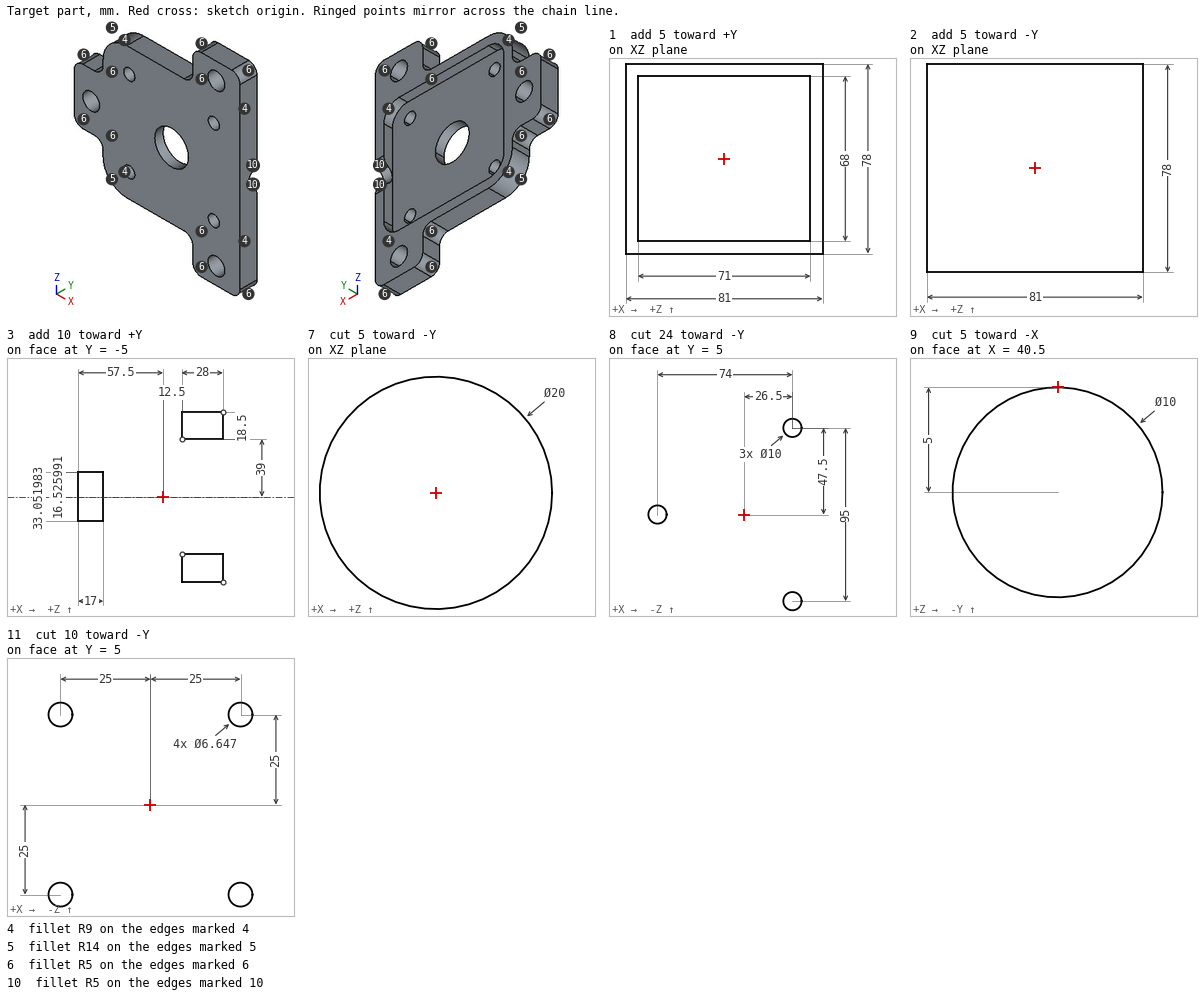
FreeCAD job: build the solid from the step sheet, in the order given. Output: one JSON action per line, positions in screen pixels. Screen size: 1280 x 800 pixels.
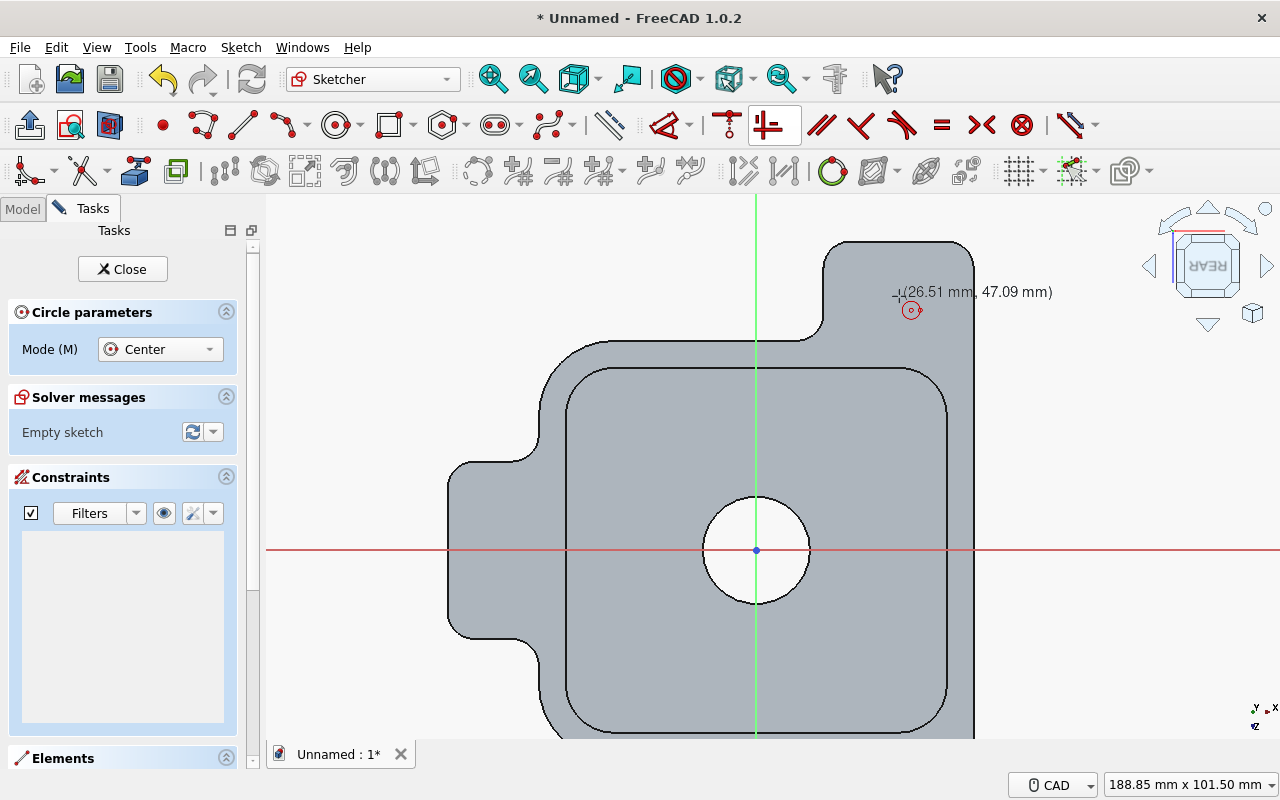
{"action": "left_click", "coordinate": [899, 295]}
{"action": "left_click", "coordinate": [918, 276]}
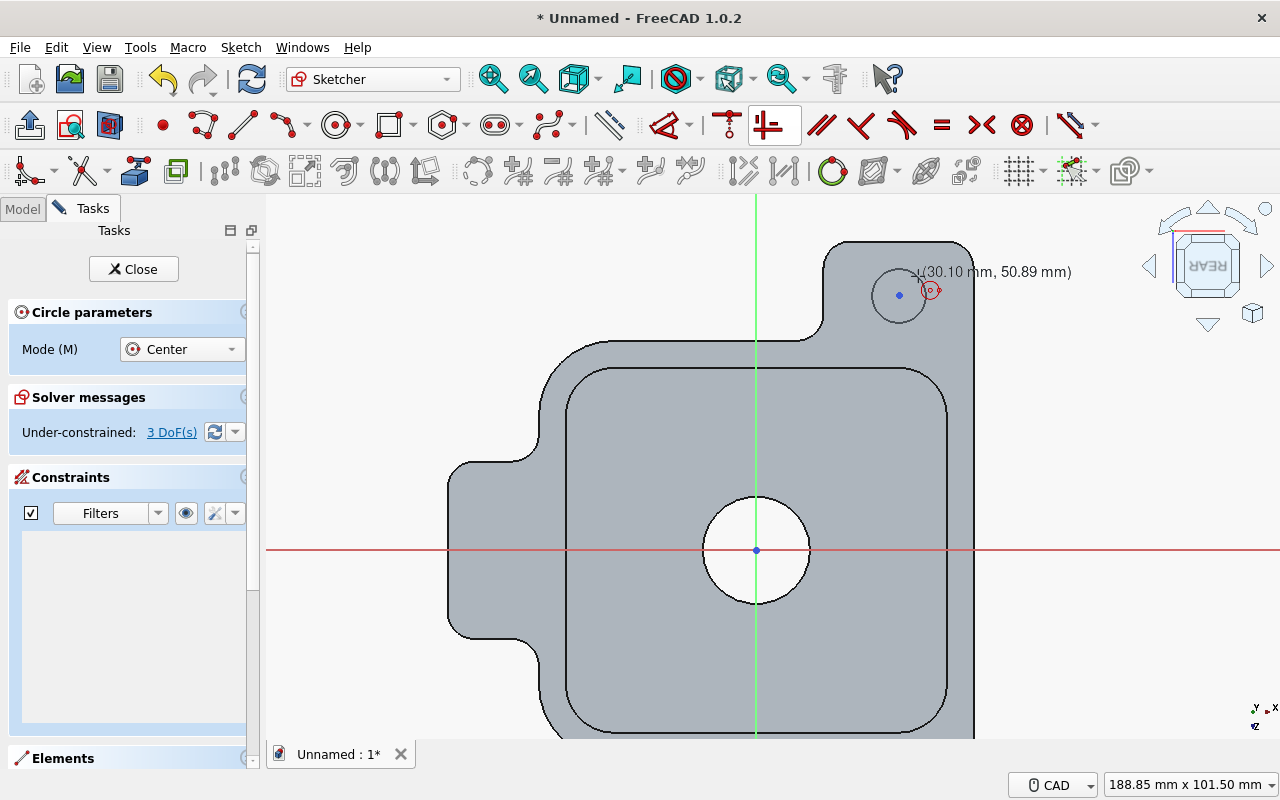
{"action": "scroll", "coordinate": [714, 296], "scroll_direction": "down", "scroll_amount": 2}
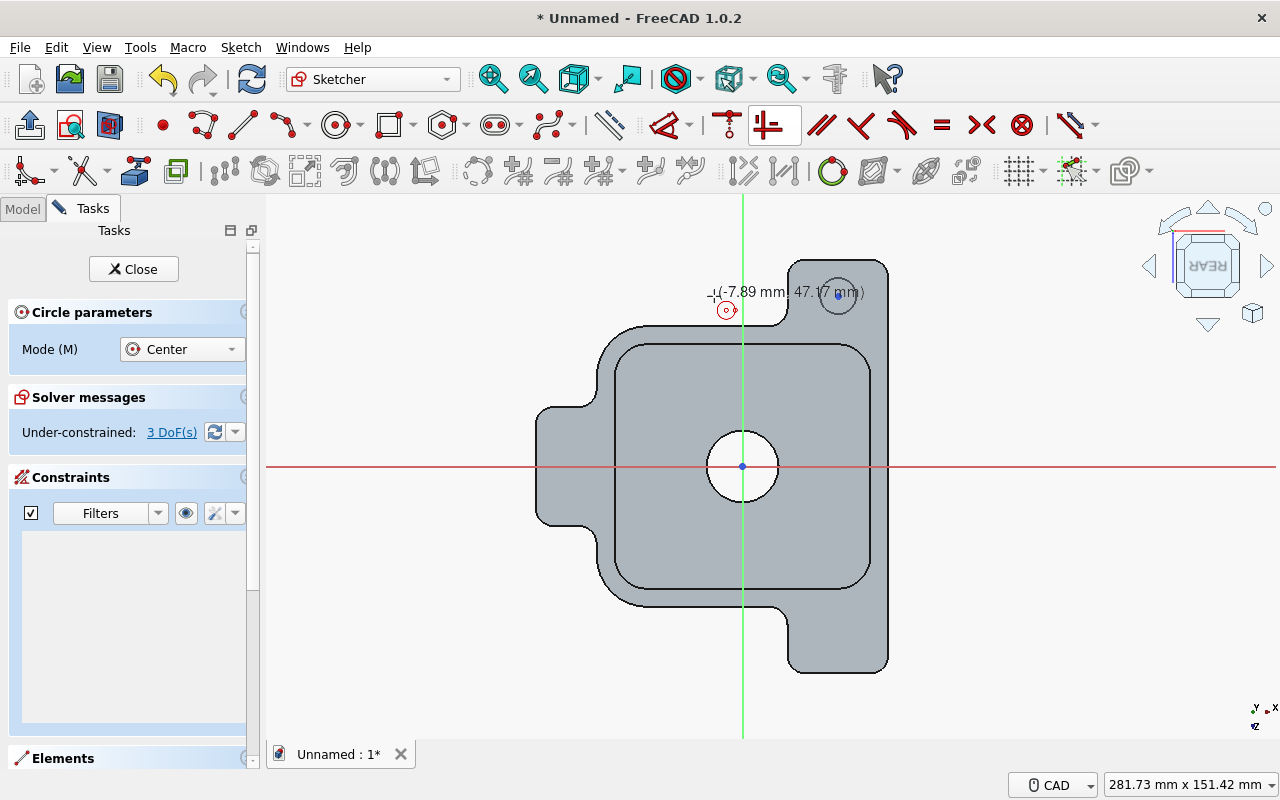
{"action": "scroll", "coordinate": [838, 637], "scroll_direction": "up", "scroll_amount": 2}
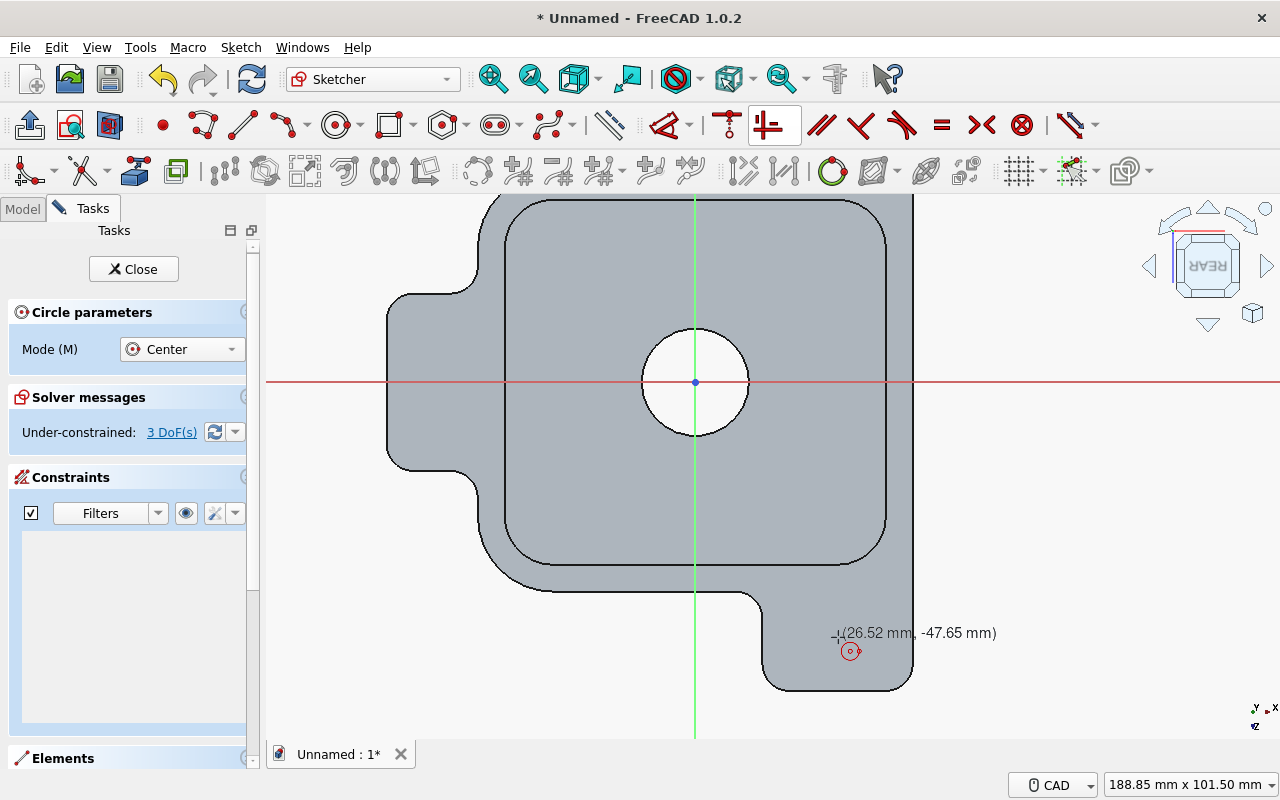
{"action": "left_click", "coordinate": [838, 637]}
{"action": "left_click", "coordinate": [857, 618]}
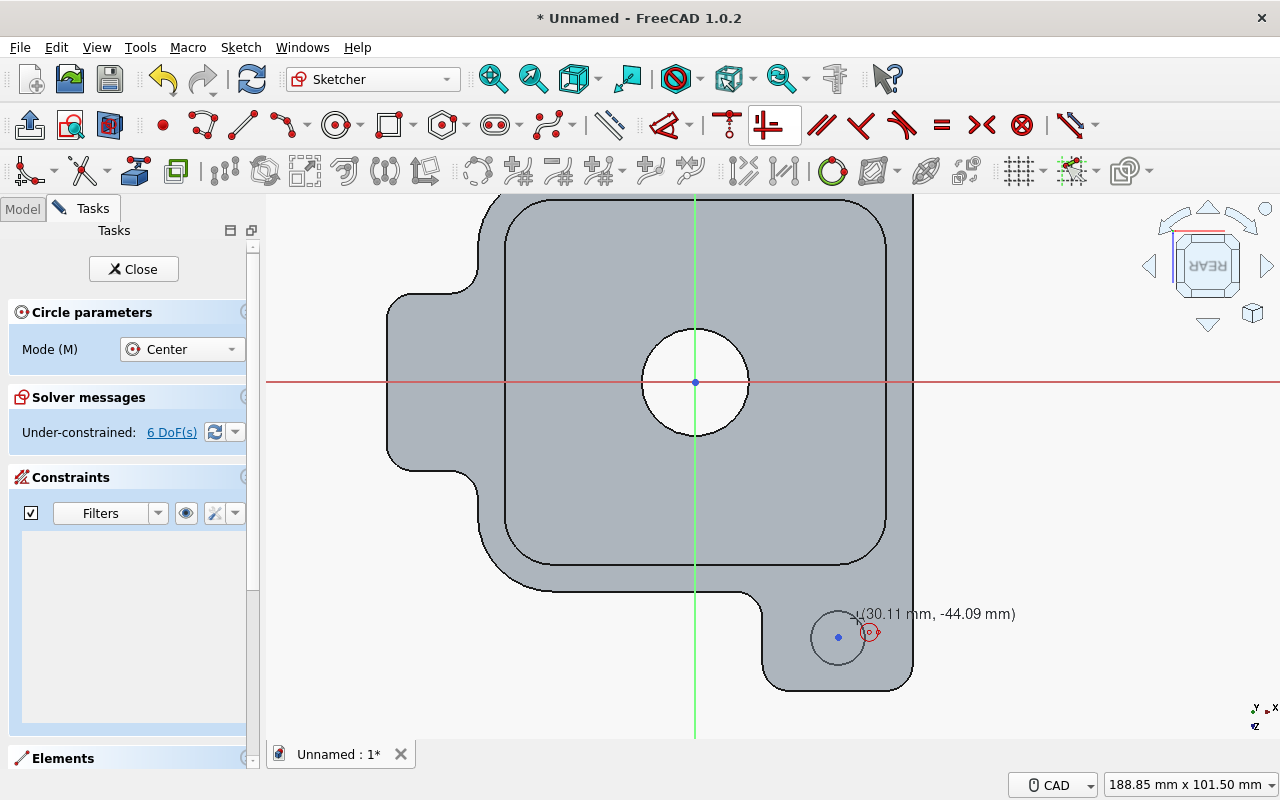
{"action": "left_click", "coordinate": [440, 382]}
{"action": "left_click", "coordinate": [459, 363]}
{"action": "key", "text": "Escape"}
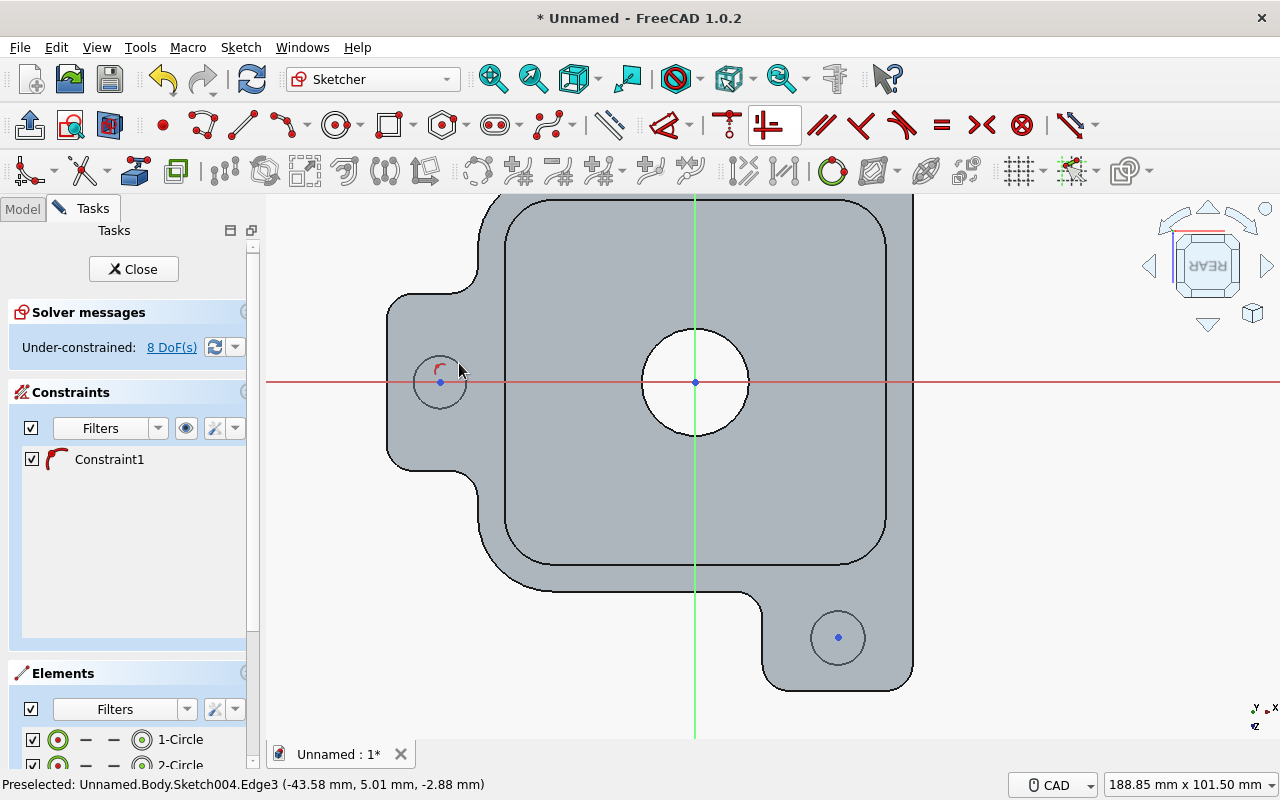
{"action": "scroll", "coordinate": [838, 638], "scroll_direction": "down", "scroll_amount": 2}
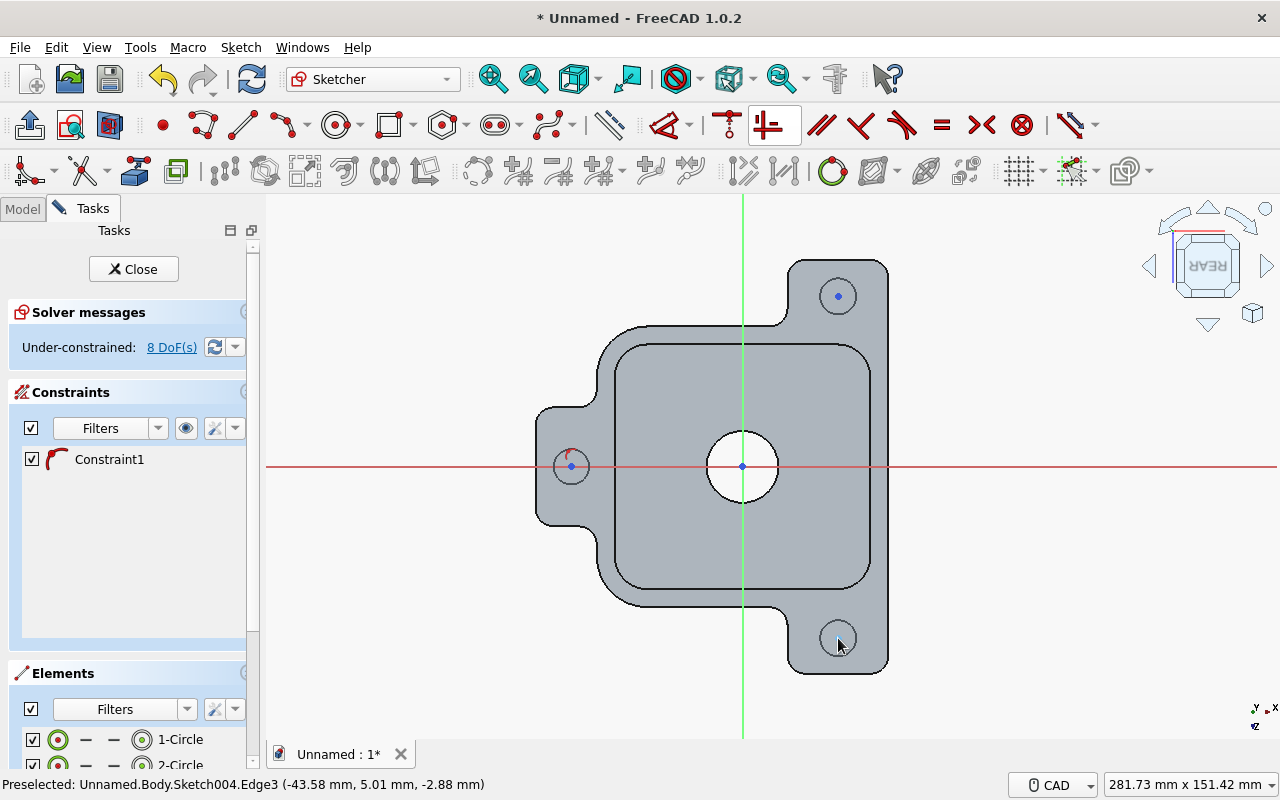
{"action": "left_click", "coordinate": [851, 284]}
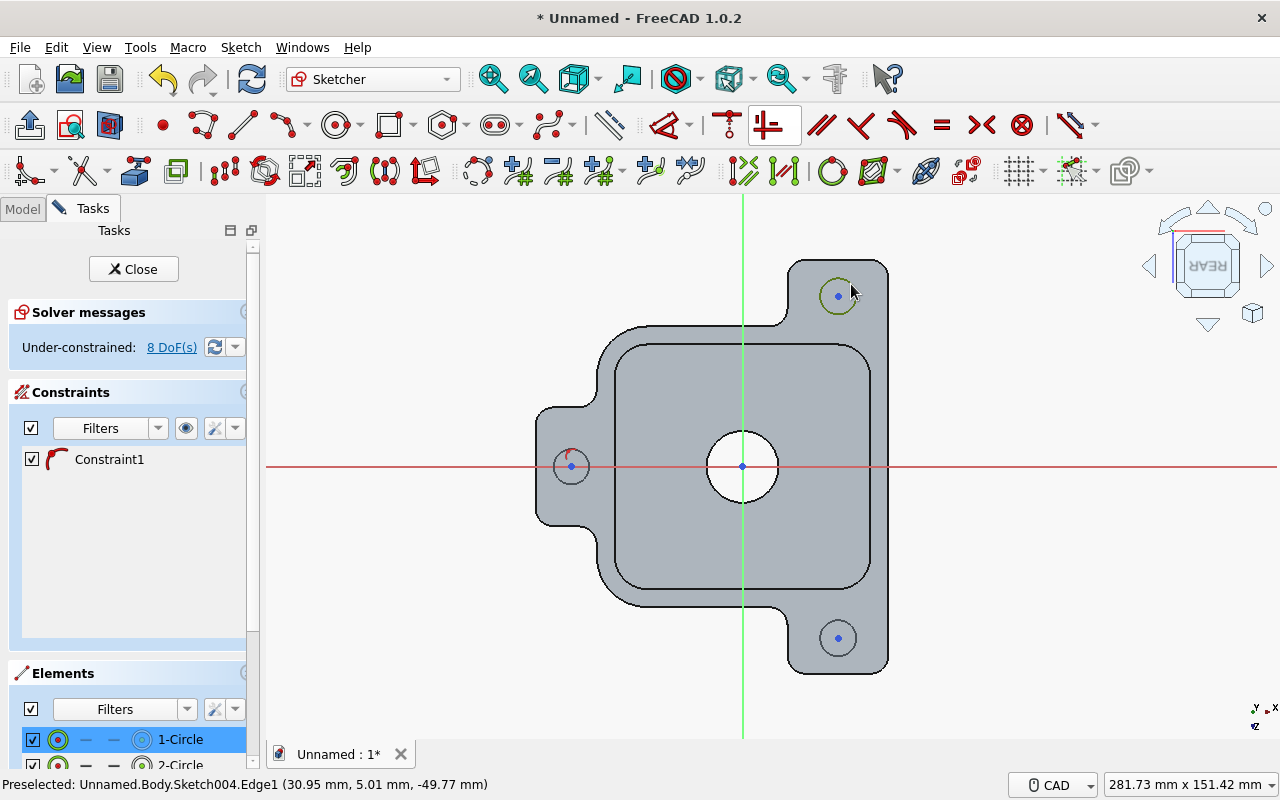
{"action": "left_click", "coordinate": [851, 625]}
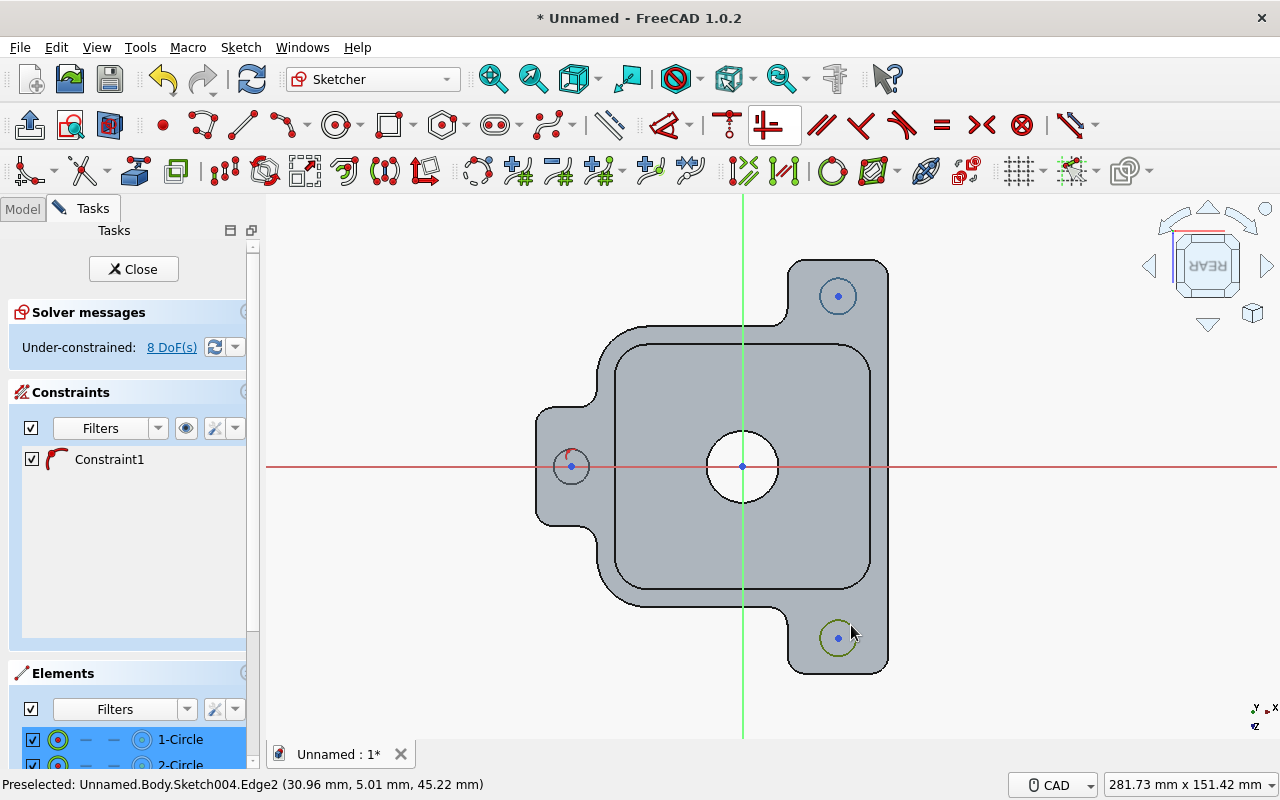
{"action": "left_click", "coordinate": [584, 454]}